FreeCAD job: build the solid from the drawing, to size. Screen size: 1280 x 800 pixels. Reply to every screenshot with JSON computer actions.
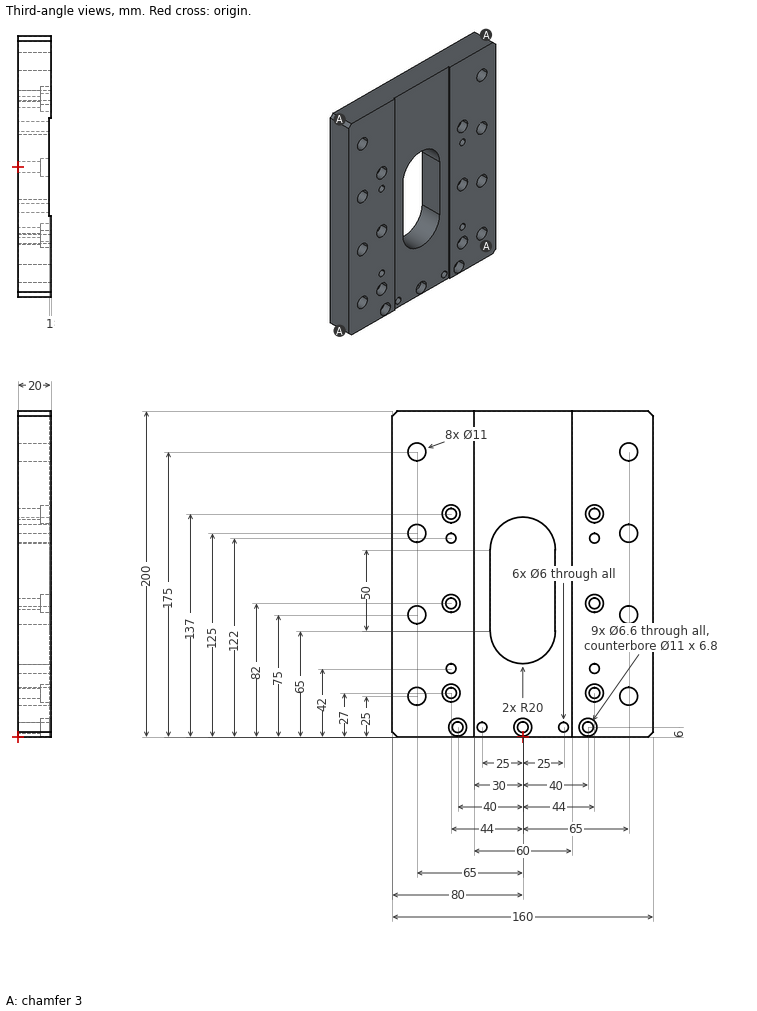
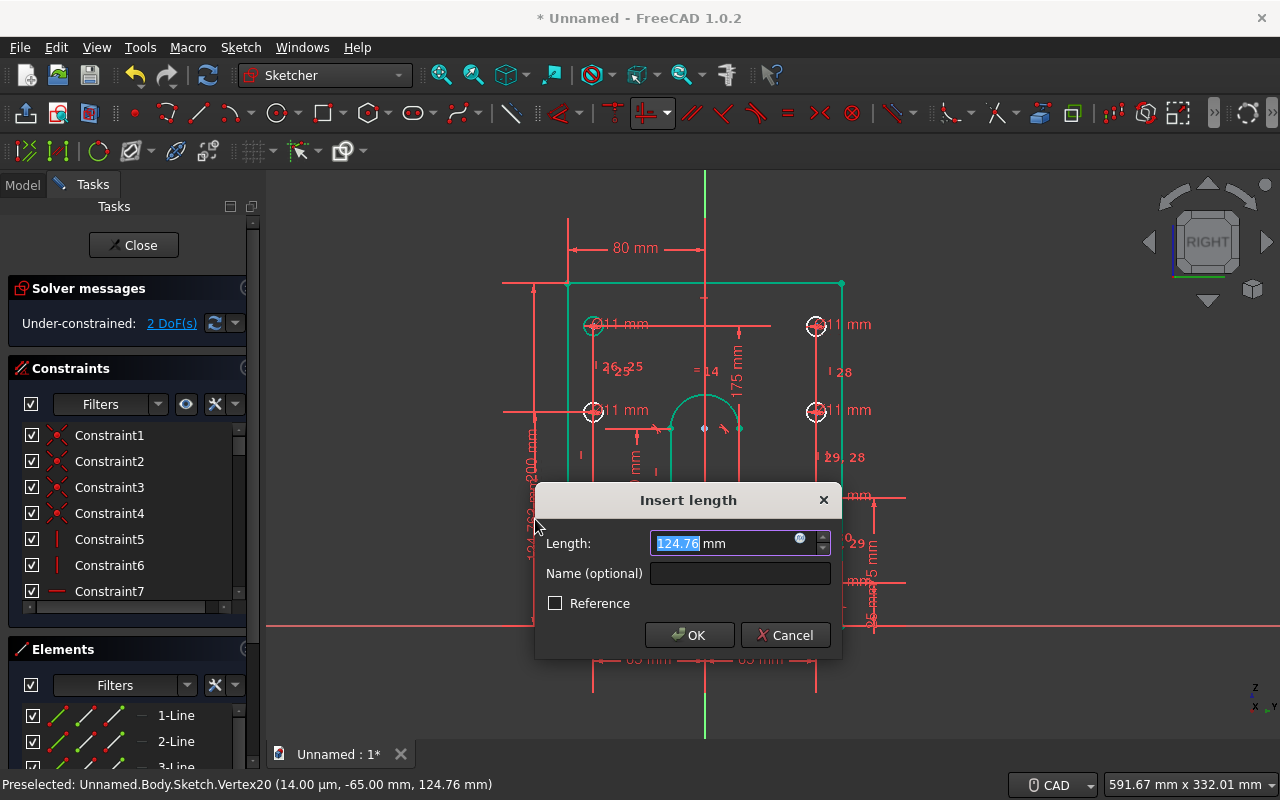
{"action": "type", "text": "125"}
{"action": "key", "text": "Return"}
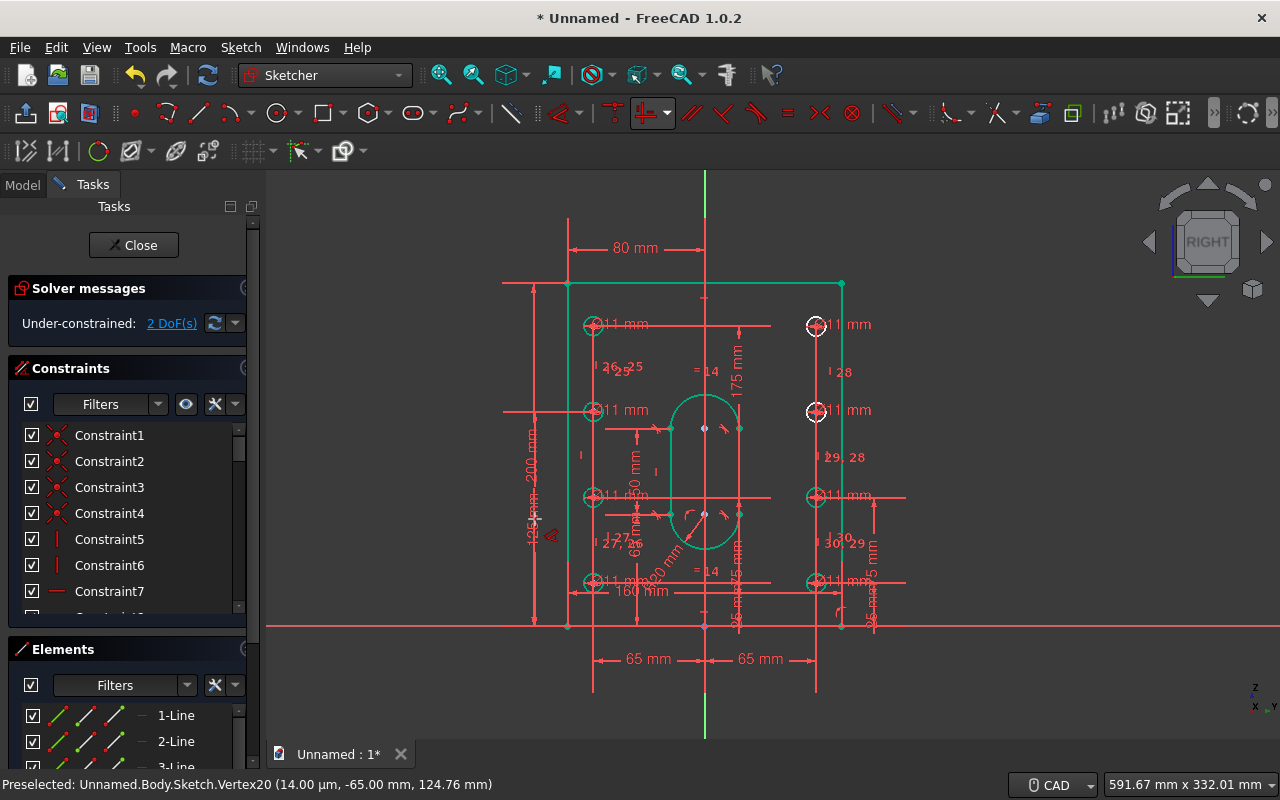
{"action": "left_click", "coordinate": [816, 327]}
{"action": "left_click", "coordinate": [874, 476]}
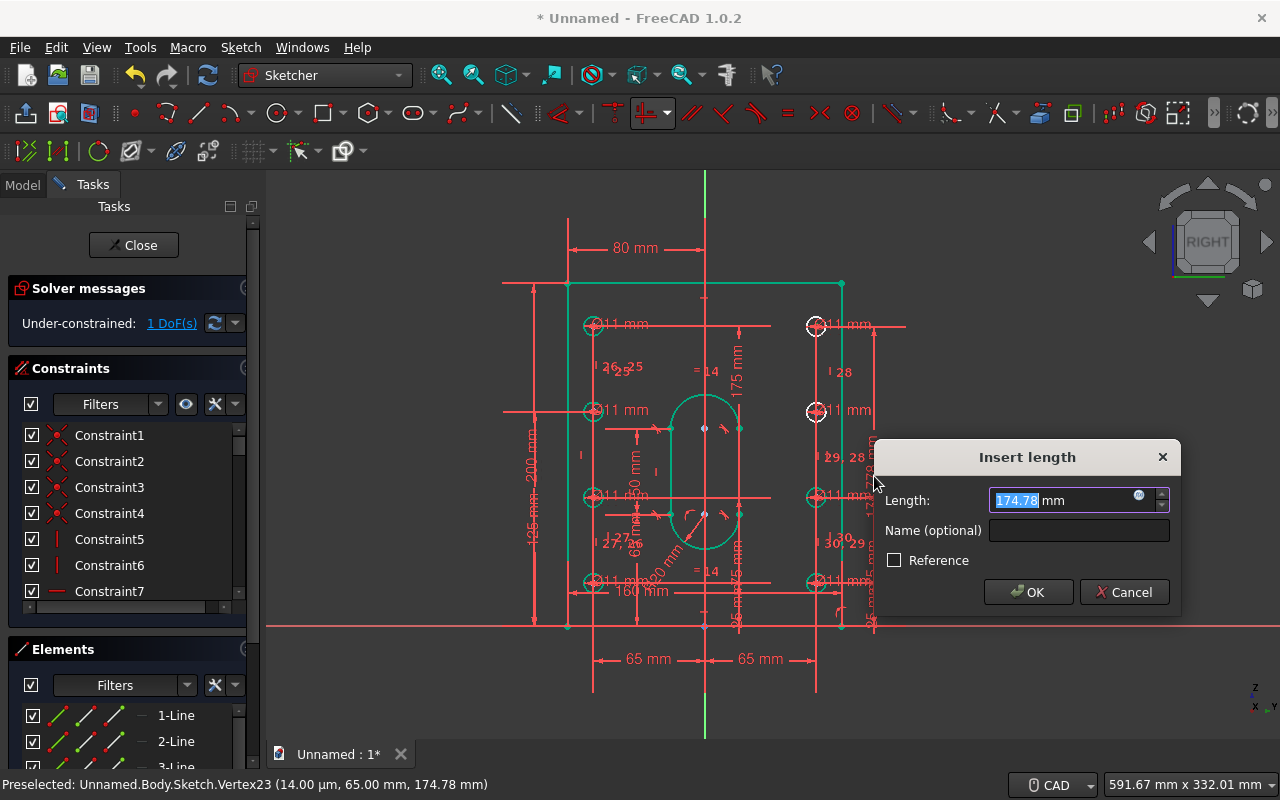
{"action": "type", "text": "175"}
{"action": "key", "text": "Return"}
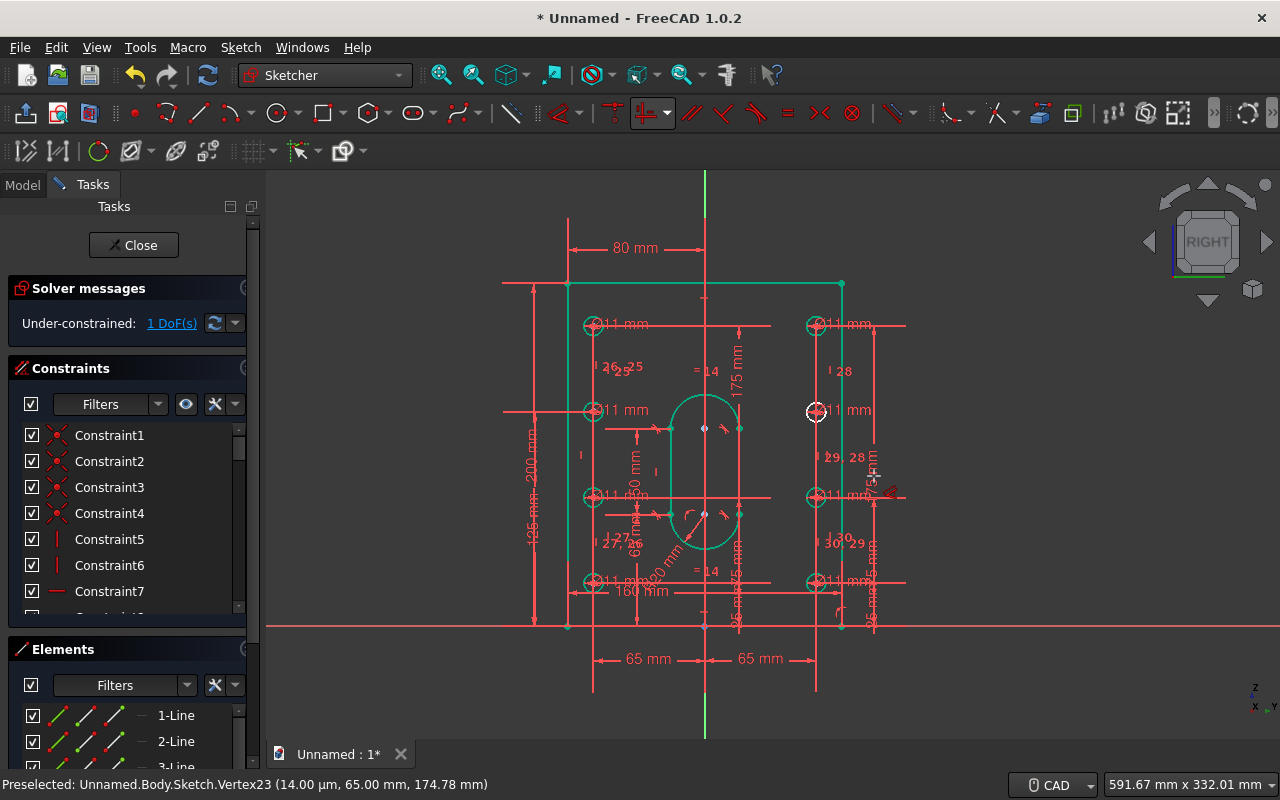
{"action": "left_click", "coordinate": [816, 412]}
{"action": "left_click", "coordinate": [874, 519]}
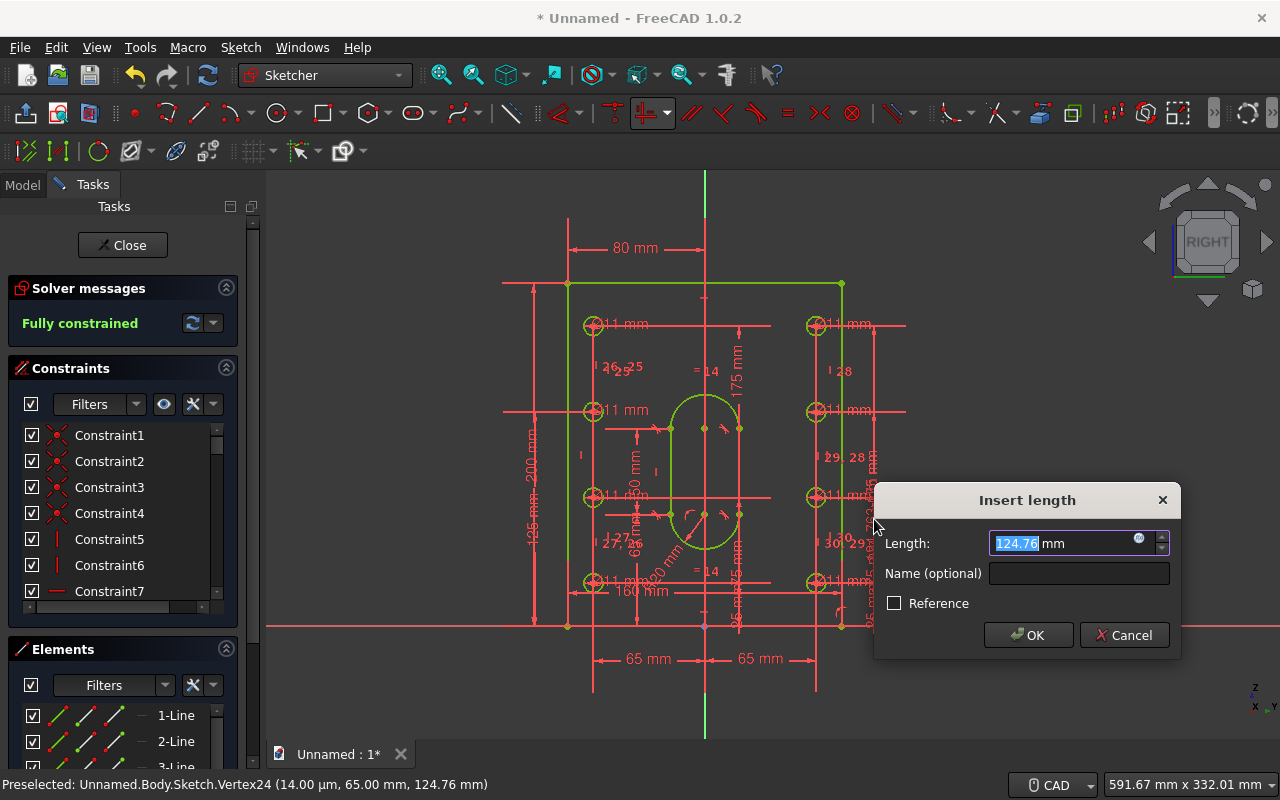
{"action": "type", "text": "125"}
{"action": "key", "text": "Return"}
{"action": "key", "text": "Escape"}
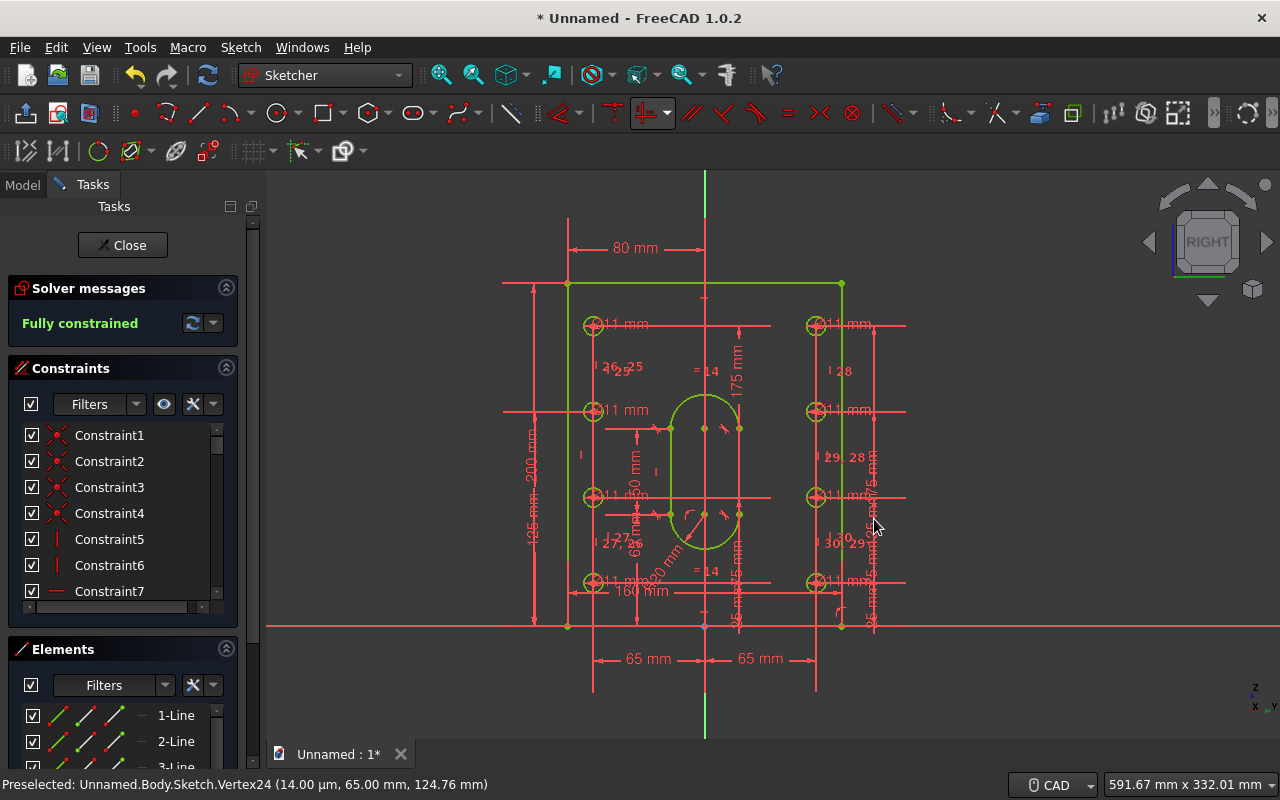
{"action": "left_click", "coordinate": [123, 245]}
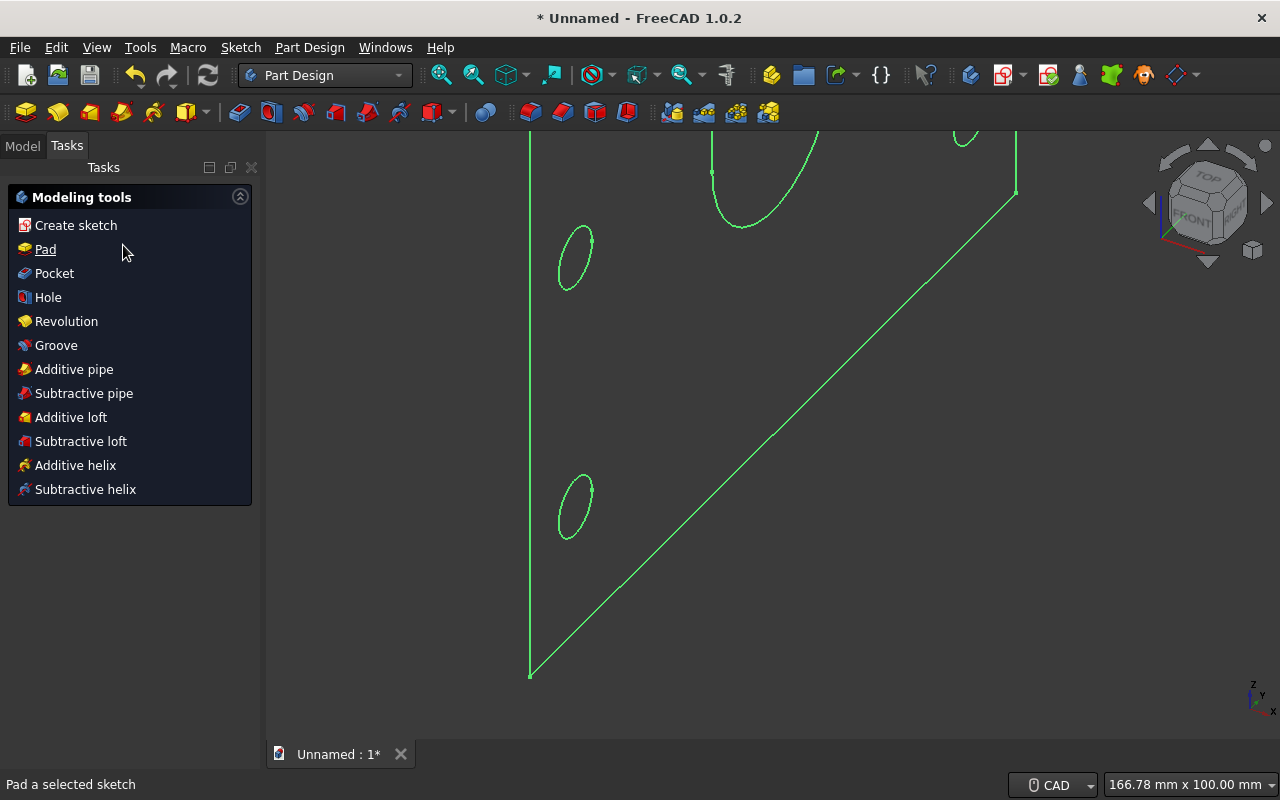
{"action": "left_click", "coordinate": [26, 112]}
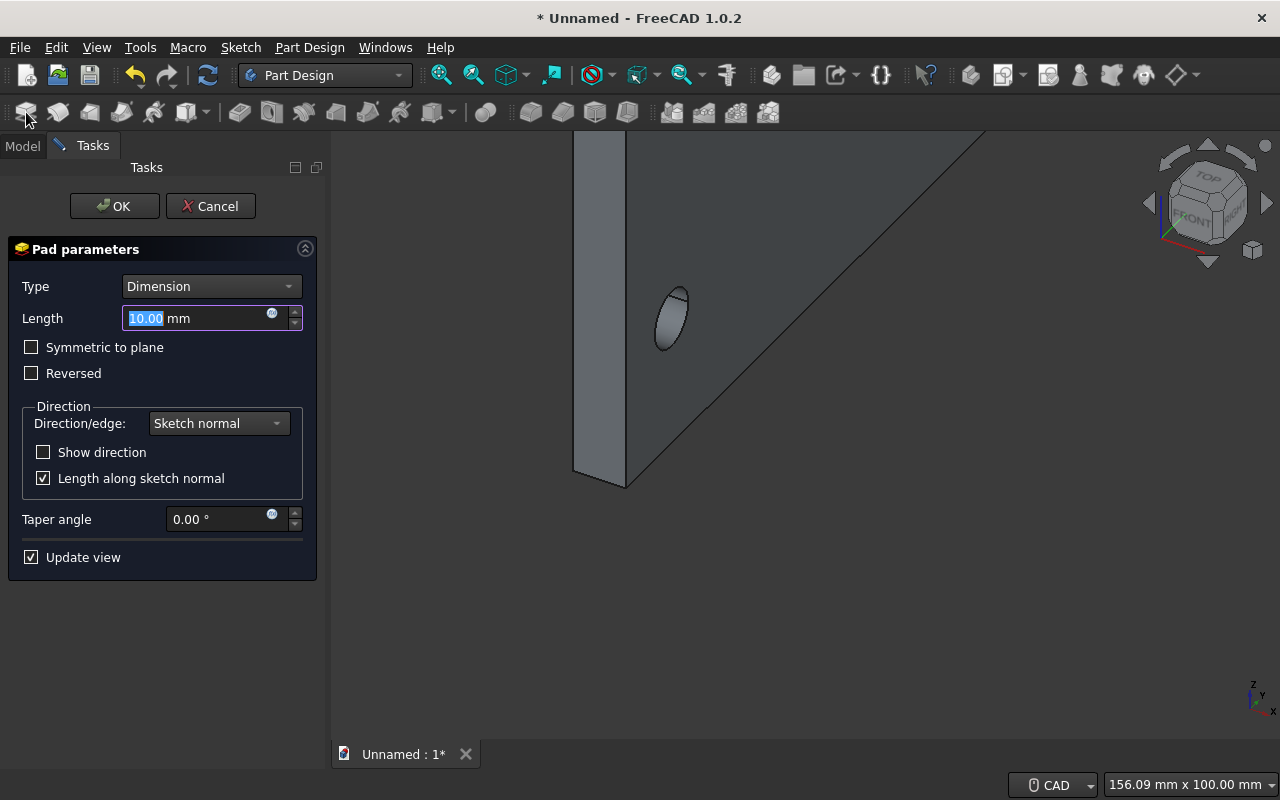
{"action": "type", "text": "20"}
{"action": "key", "text": "Tab"}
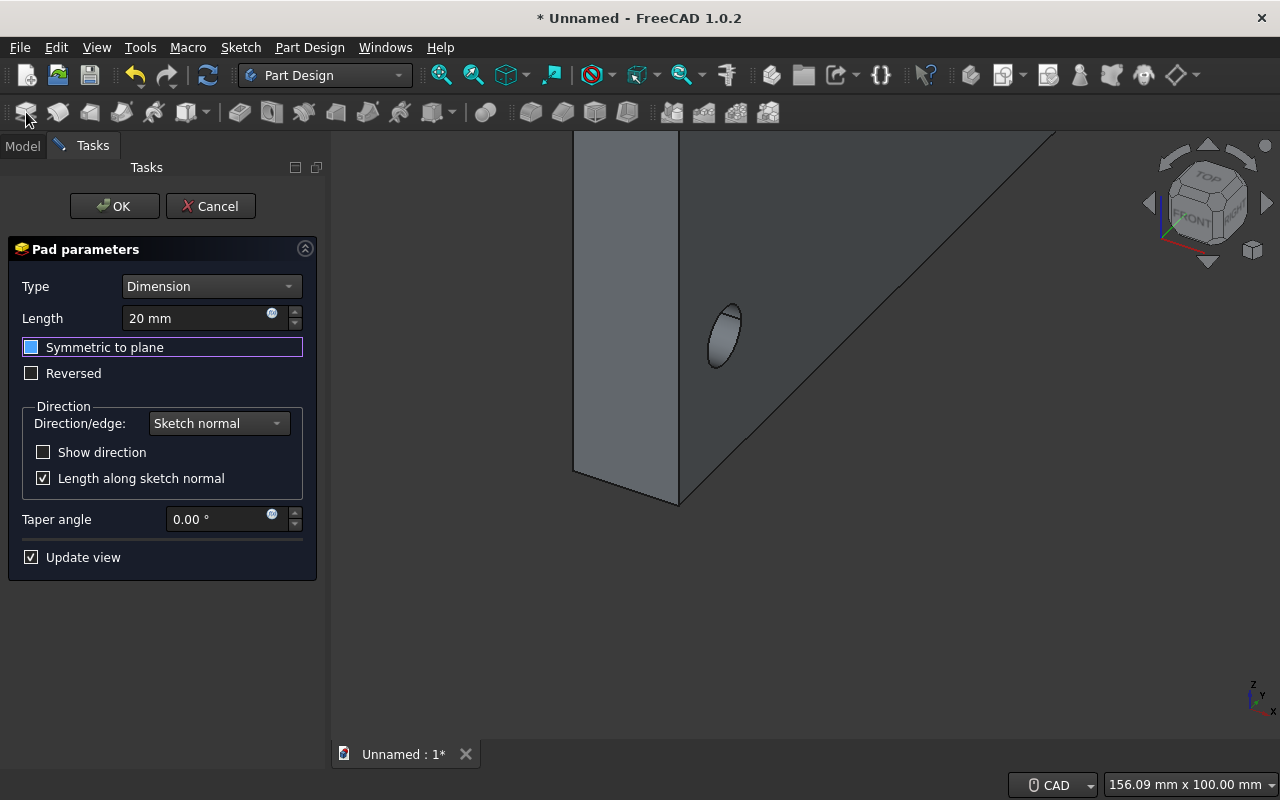
{"action": "left_click", "coordinate": [115, 206]}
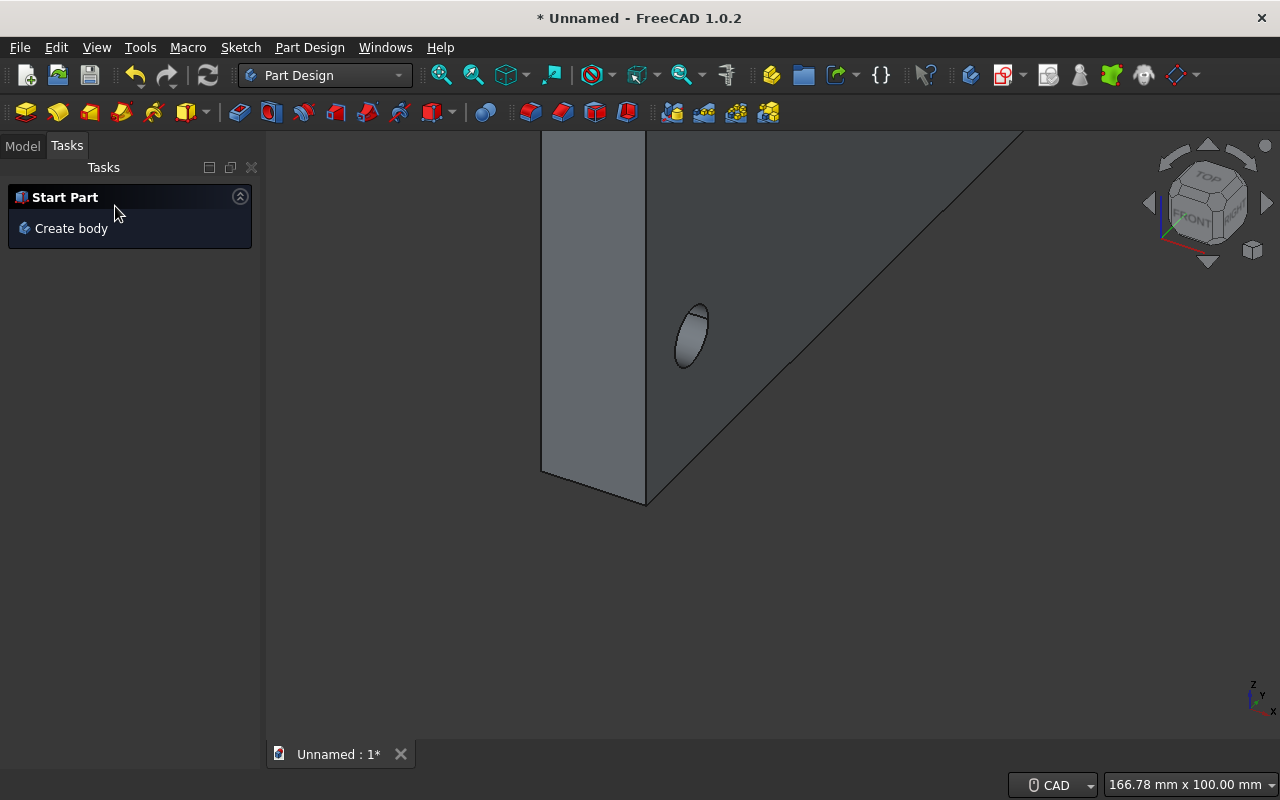
{"action": "left_click", "coordinate": [442, 76]}